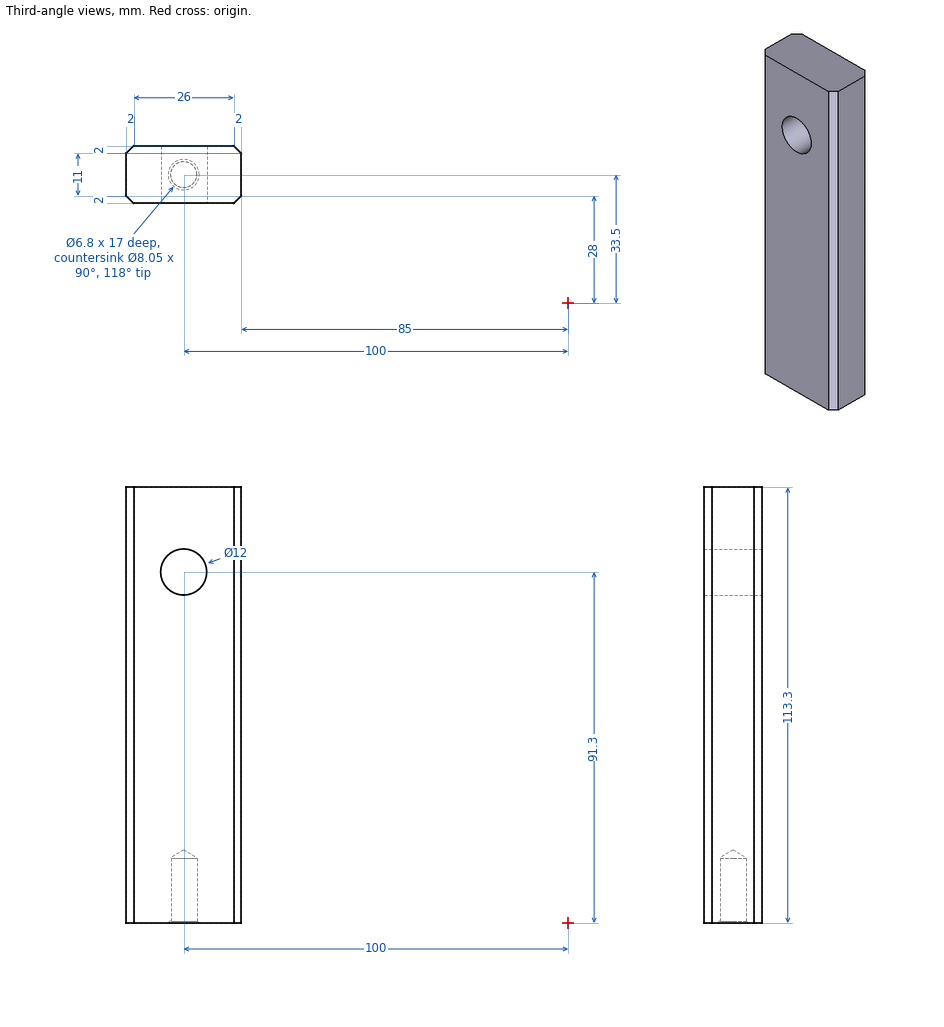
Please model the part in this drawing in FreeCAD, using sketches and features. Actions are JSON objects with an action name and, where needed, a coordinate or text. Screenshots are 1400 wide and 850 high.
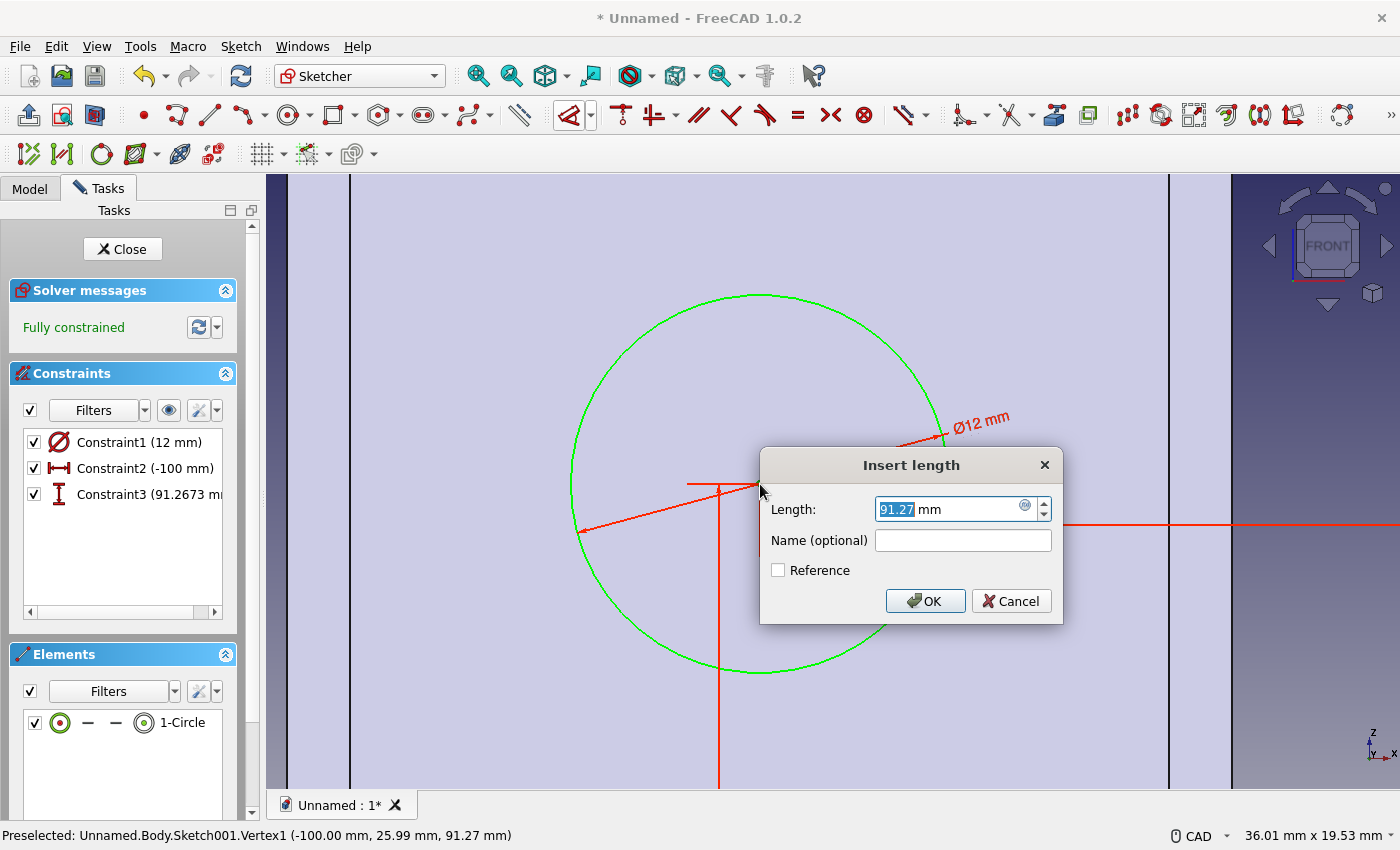
{"action": "type", "text": "91.3"}
{"action": "key", "text": "Return"}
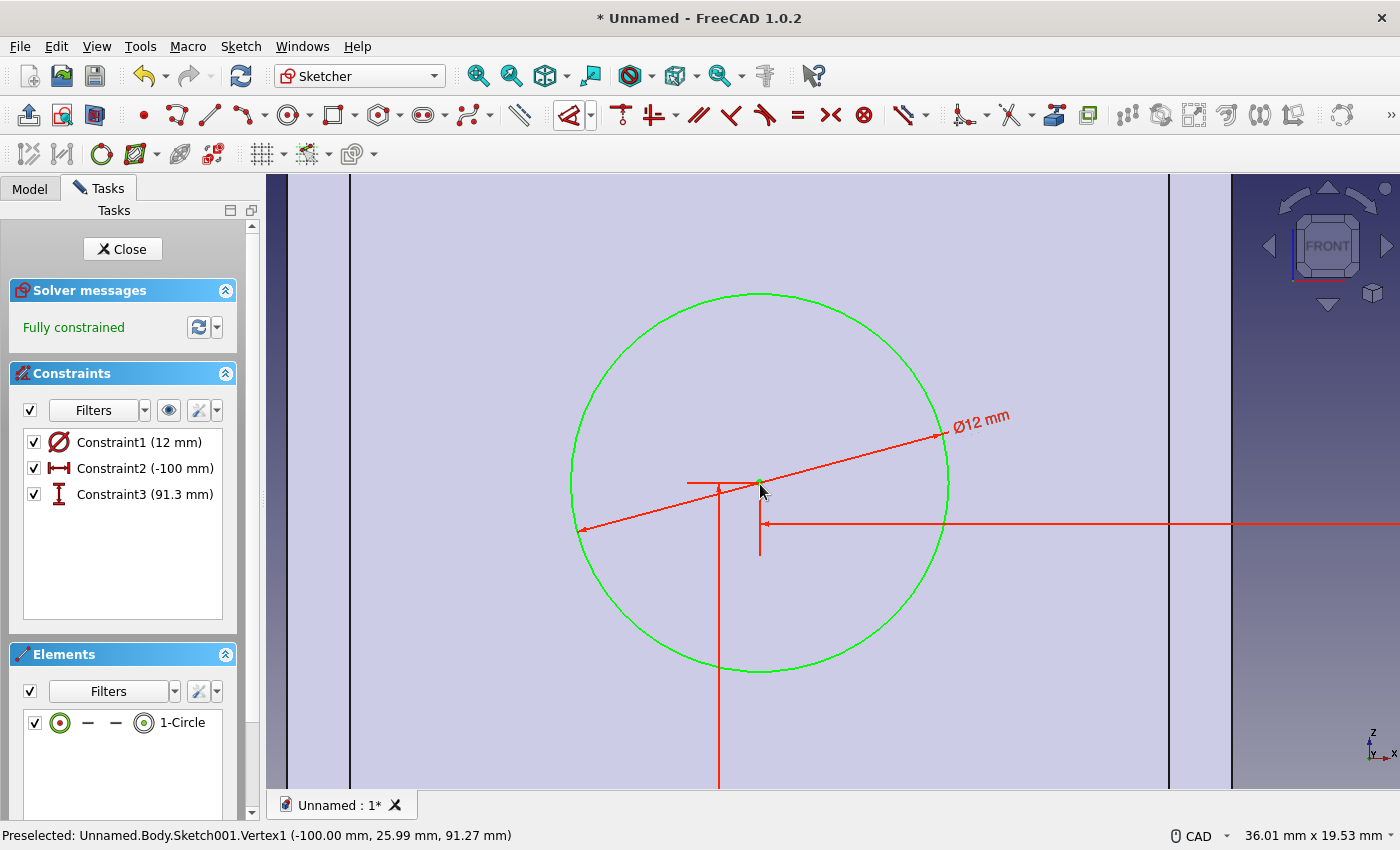
{"action": "left_click", "coordinate": [123, 249]}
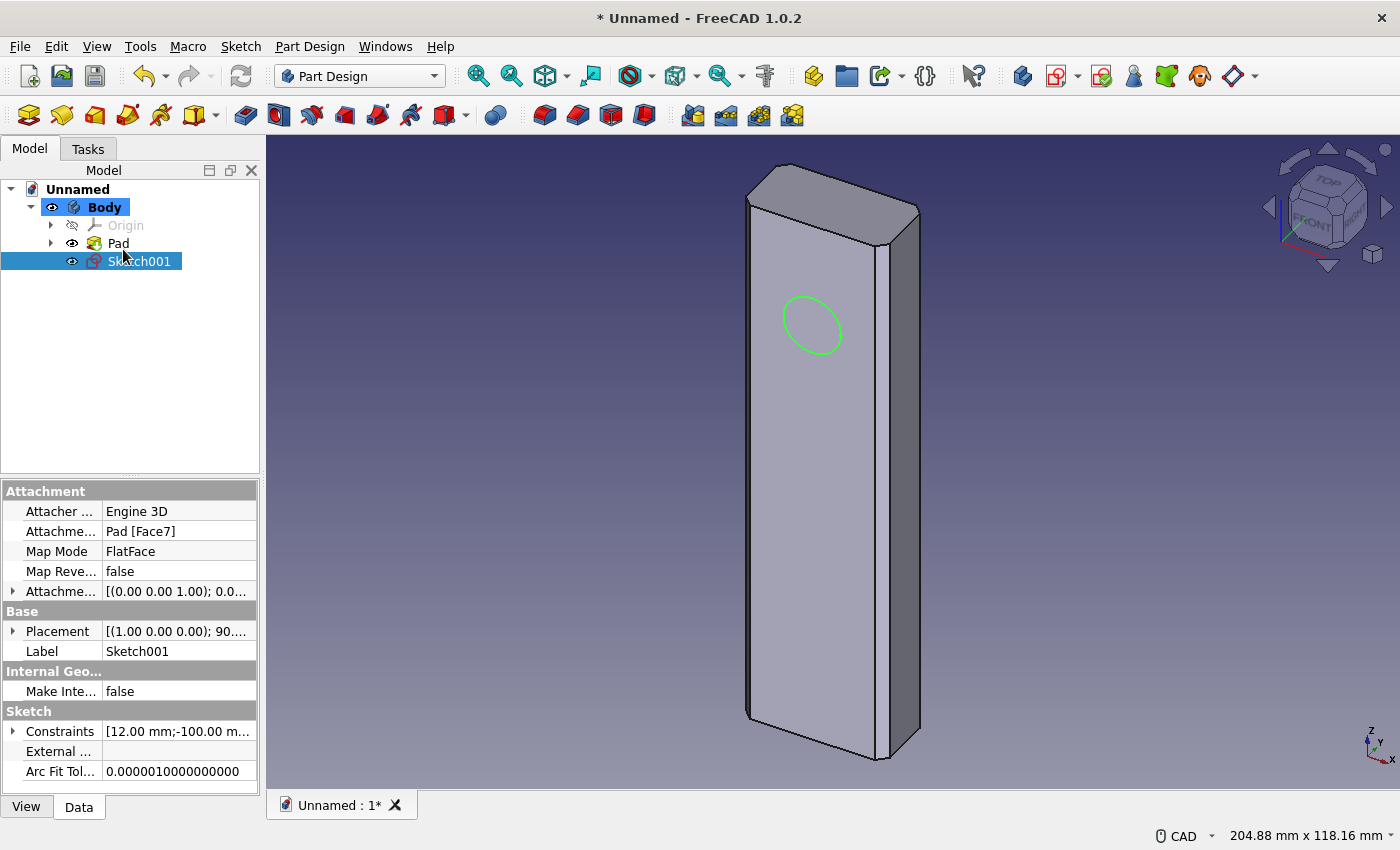
{"action": "left_click", "coordinate": [246, 116]}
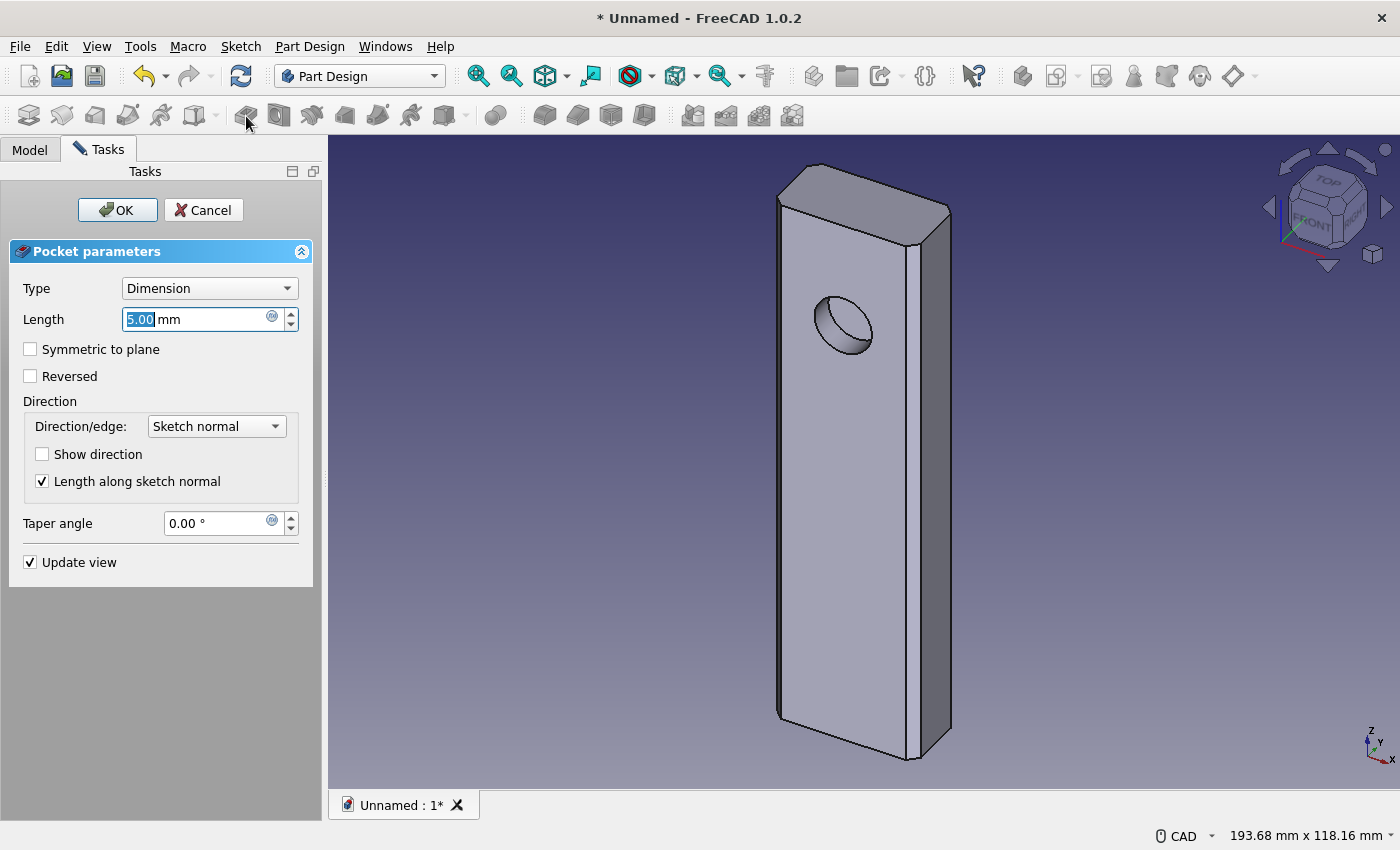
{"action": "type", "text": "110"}
{"action": "key", "text": "Tab"}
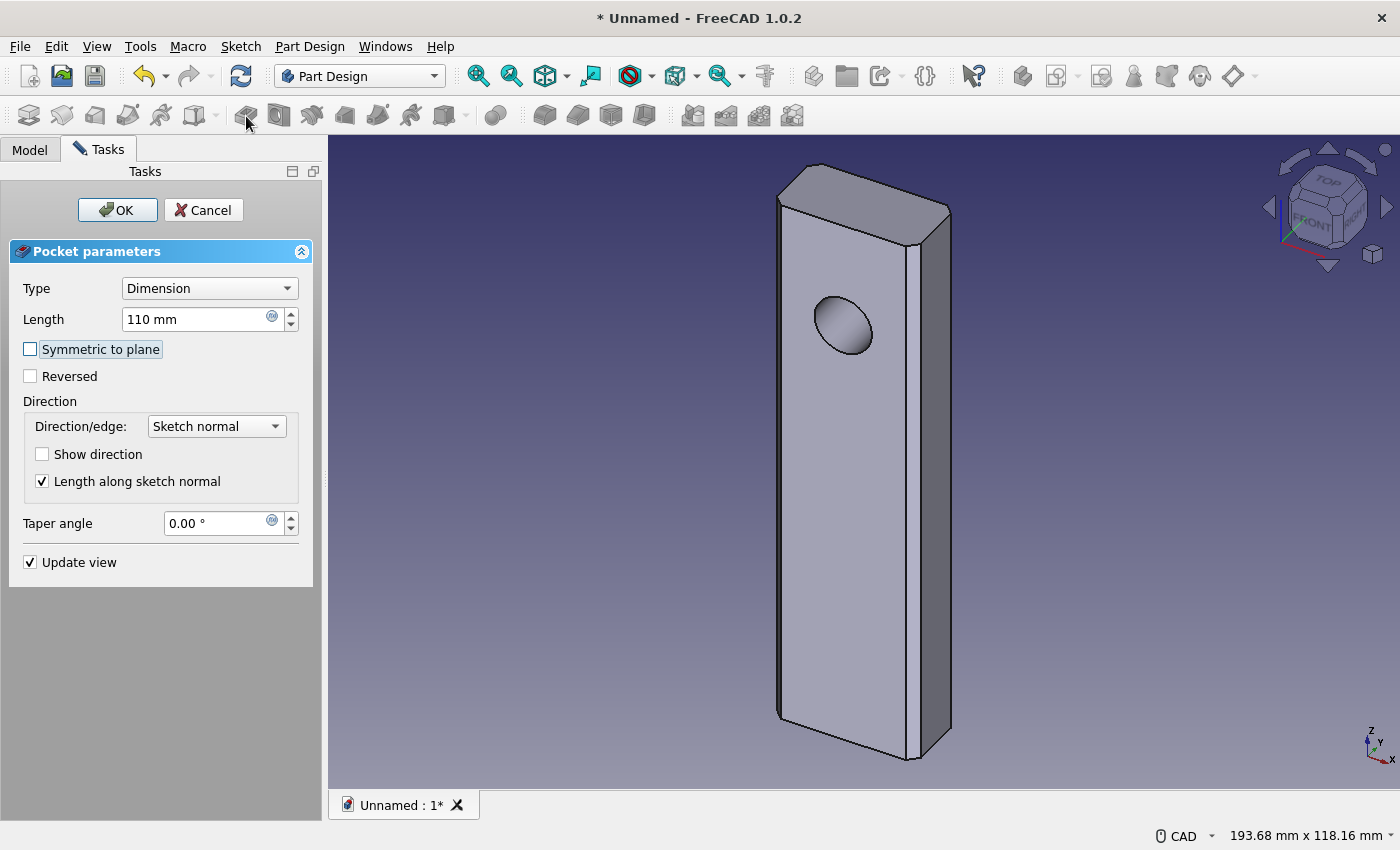
{"action": "left_click", "coordinate": [118, 210]}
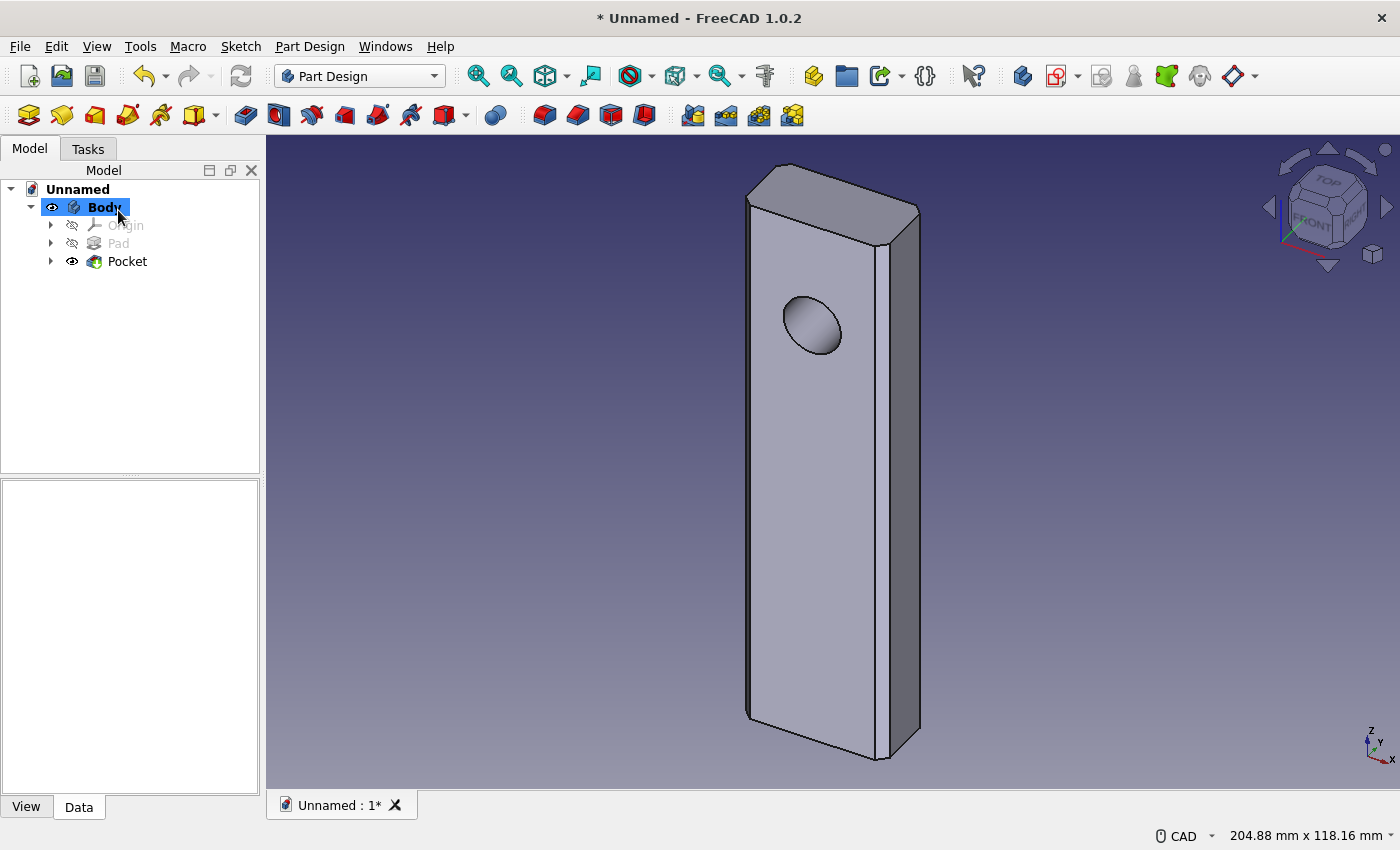
{"action": "key", "text": "5"}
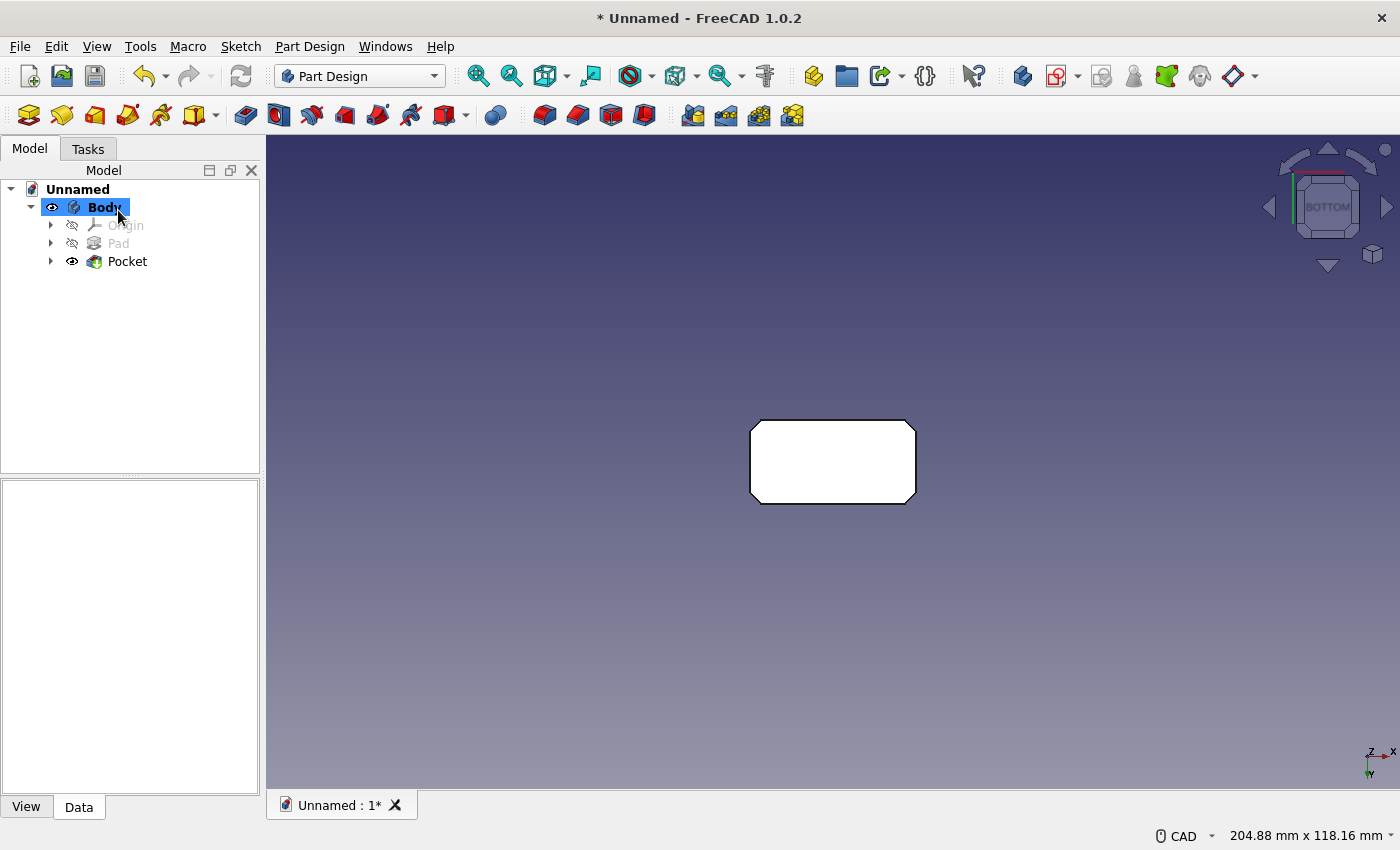
{"action": "left_click", "coordinate": [479, 76]}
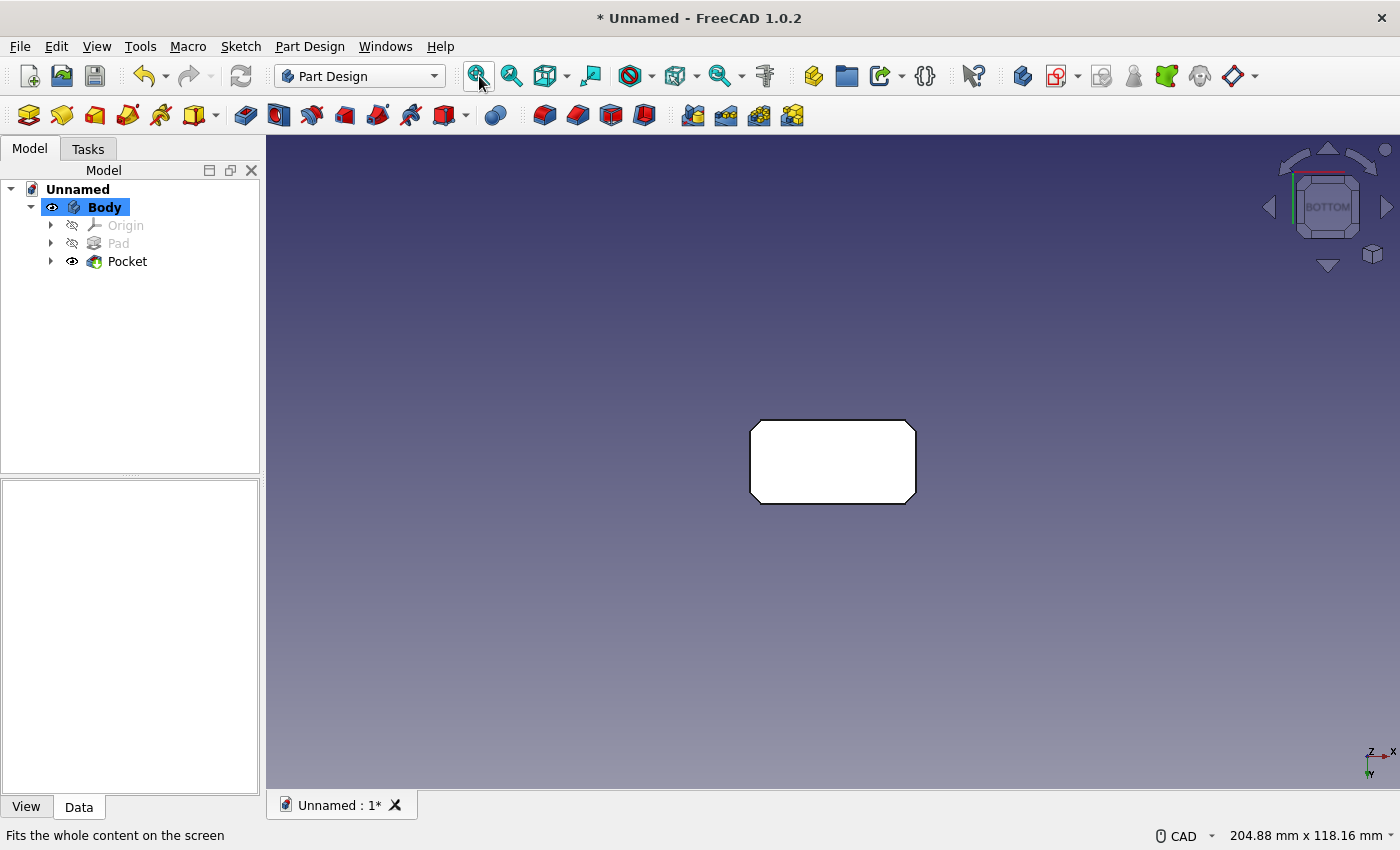
{"action": "left_click", "coordinate": [857, 461]}